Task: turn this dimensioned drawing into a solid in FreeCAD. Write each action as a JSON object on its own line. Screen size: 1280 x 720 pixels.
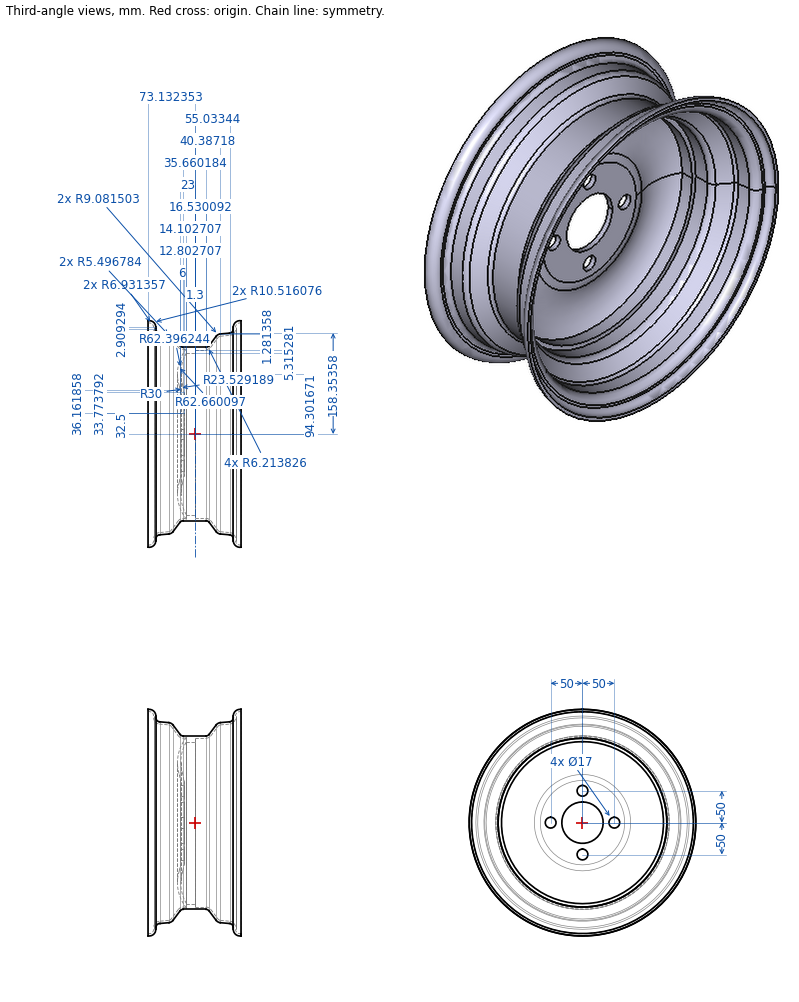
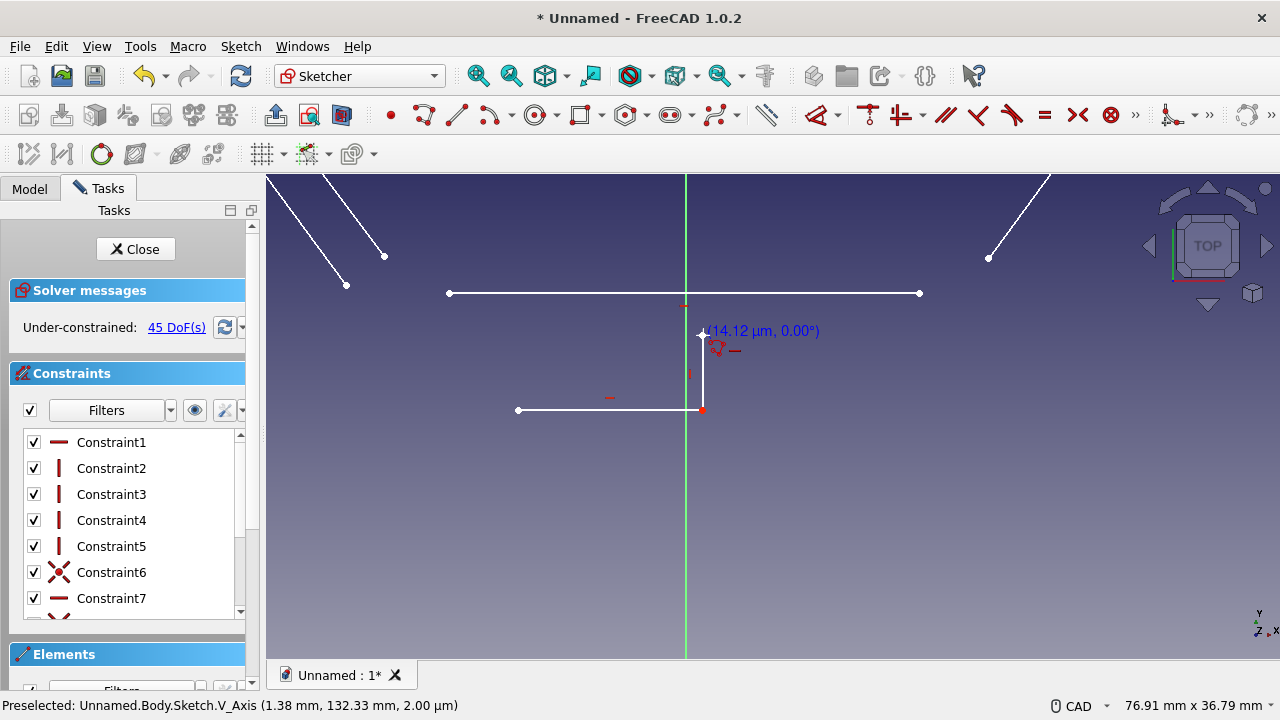
{"action": "scroll", "coordinate": [707, 339], "scroll_direction": "down", "scroll_amount": 10}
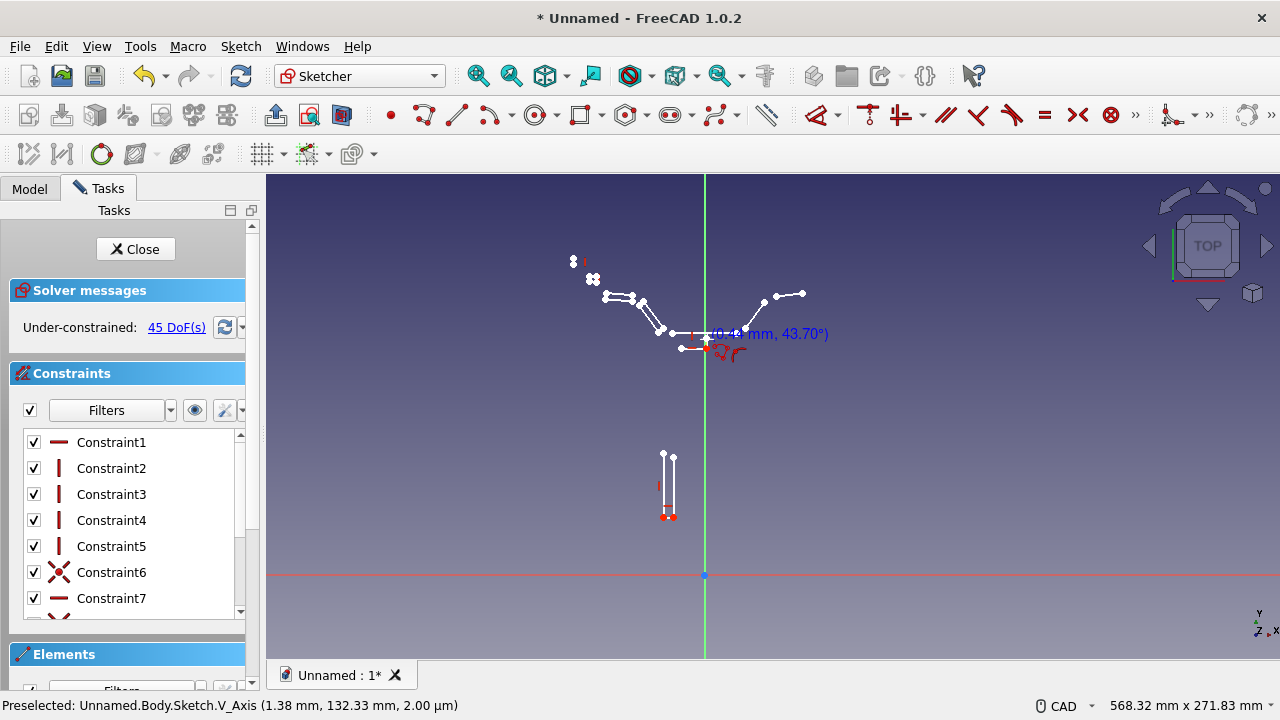
{"action": "scroll", "coordinate": [736, 339], "scroll_direction": "up", "scroll_amount": 5}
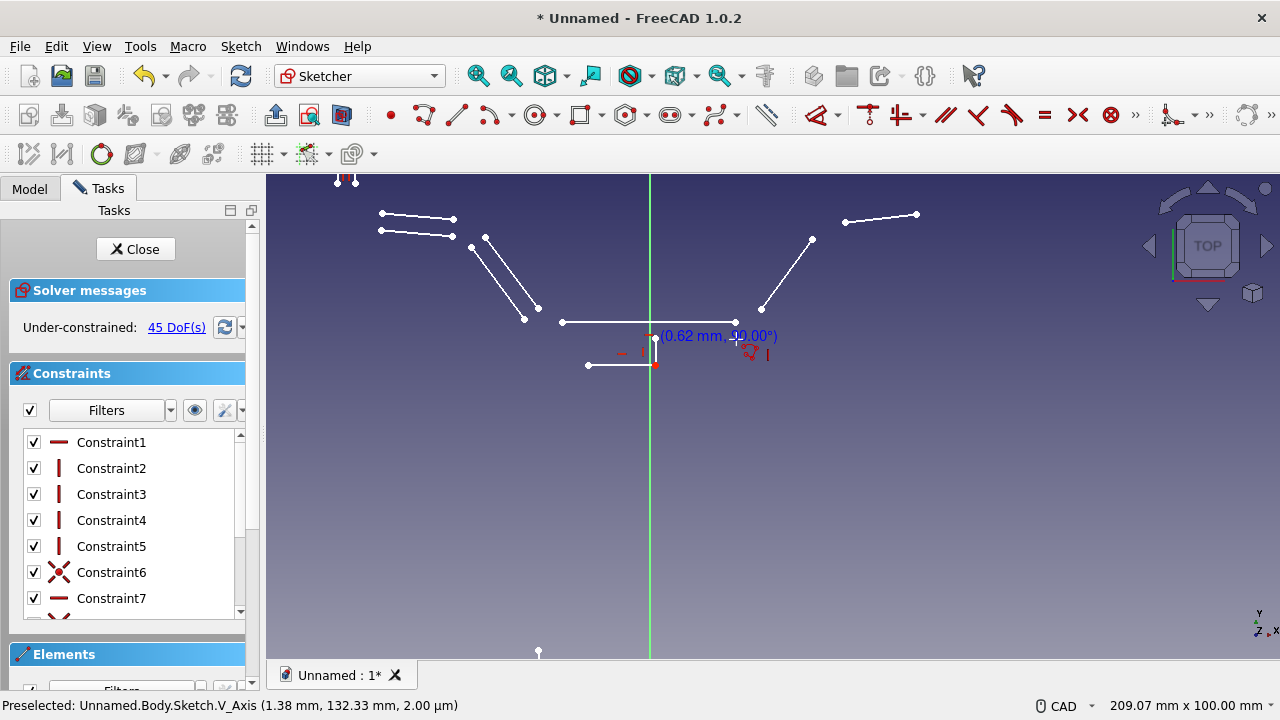
{"action": "left_click", "coordinate": [736, 338]}
{"action": "right_click", "coordinate": [736, 338]}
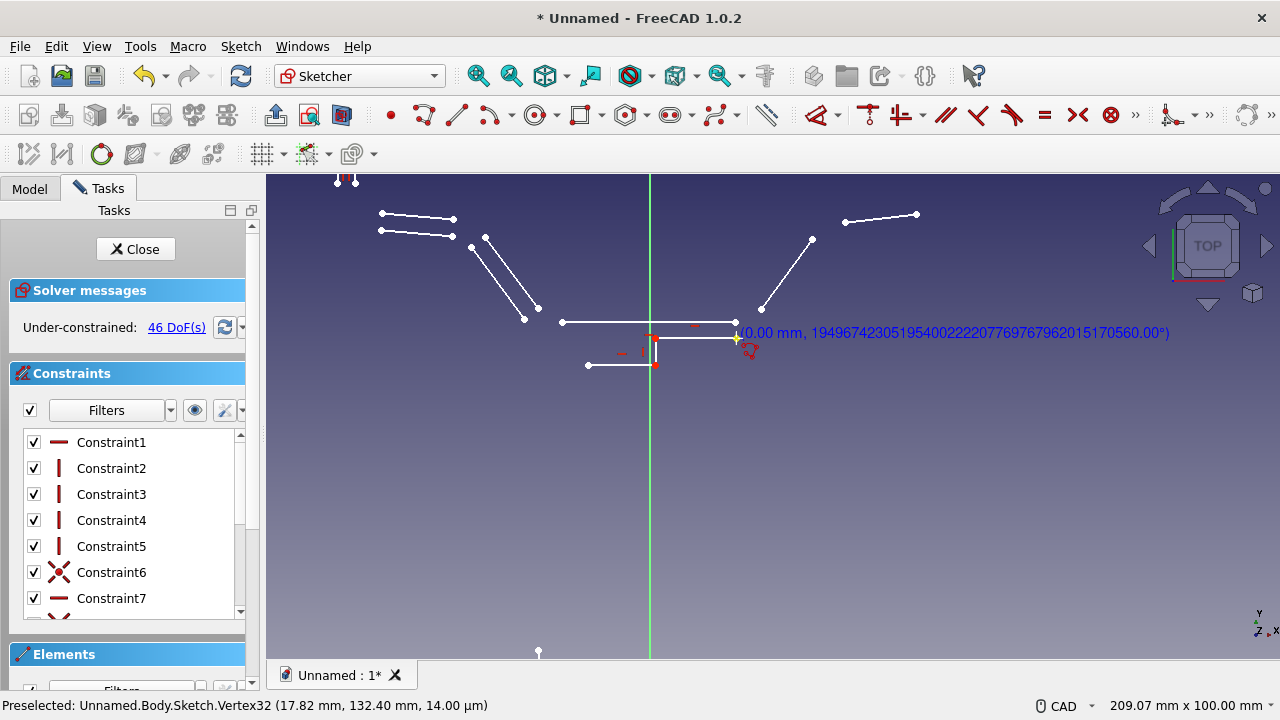
{"action": "left_click", "coordinate": [457, 116]}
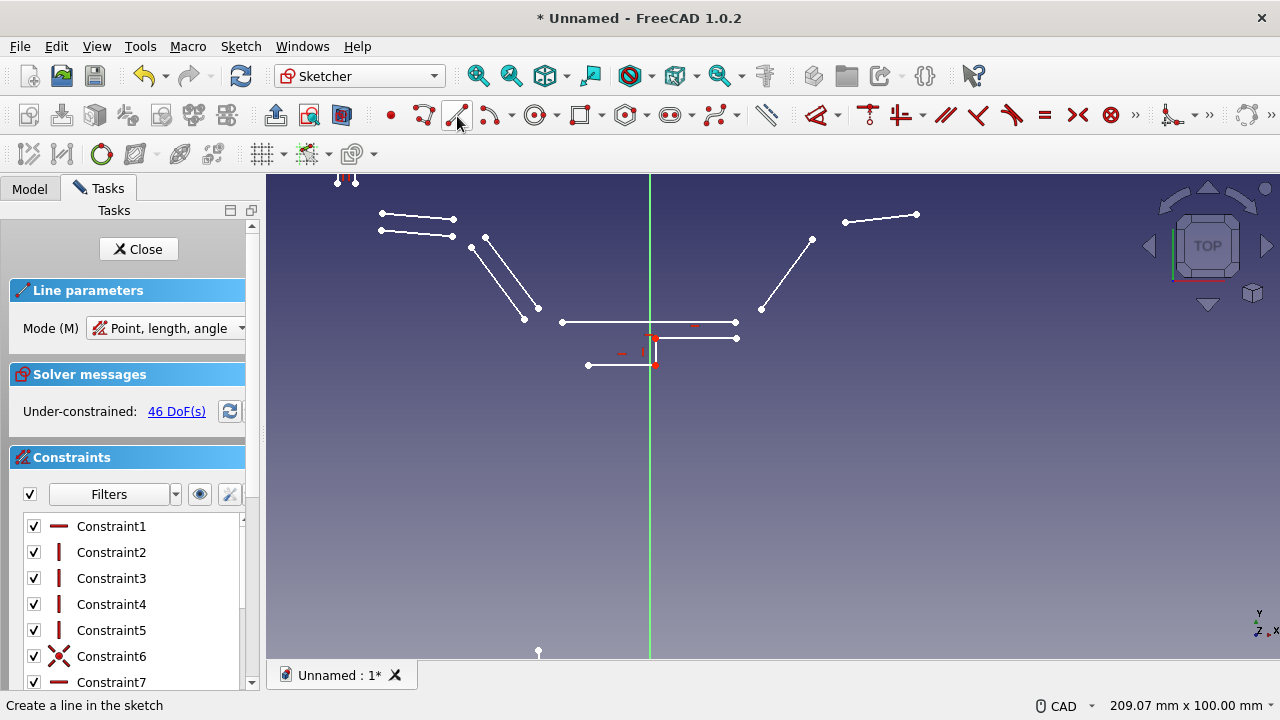
{"action": "left_click", "coordinate": [774, 318]}
{"action": "left_click", "coordinate": [828, 246]}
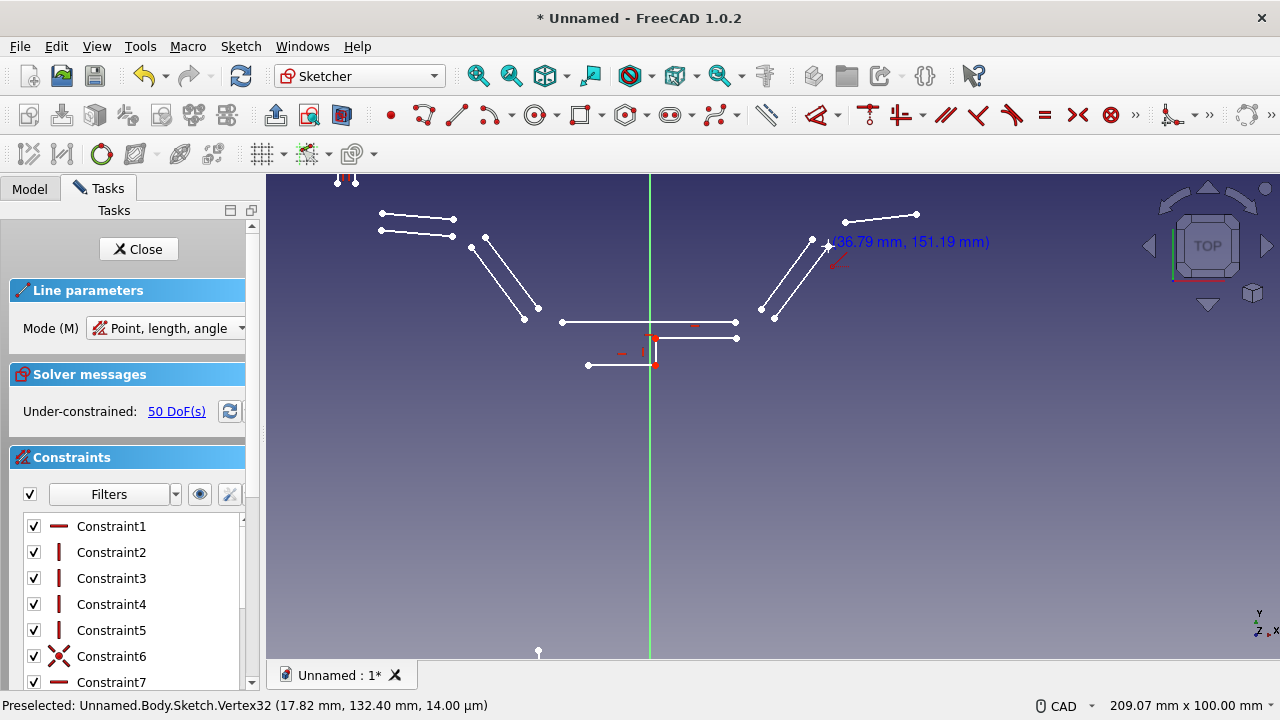
{"action": "left_click", "coordinate": [847, 236]}
{"action": "left_click", "coordinate": [918, 230]}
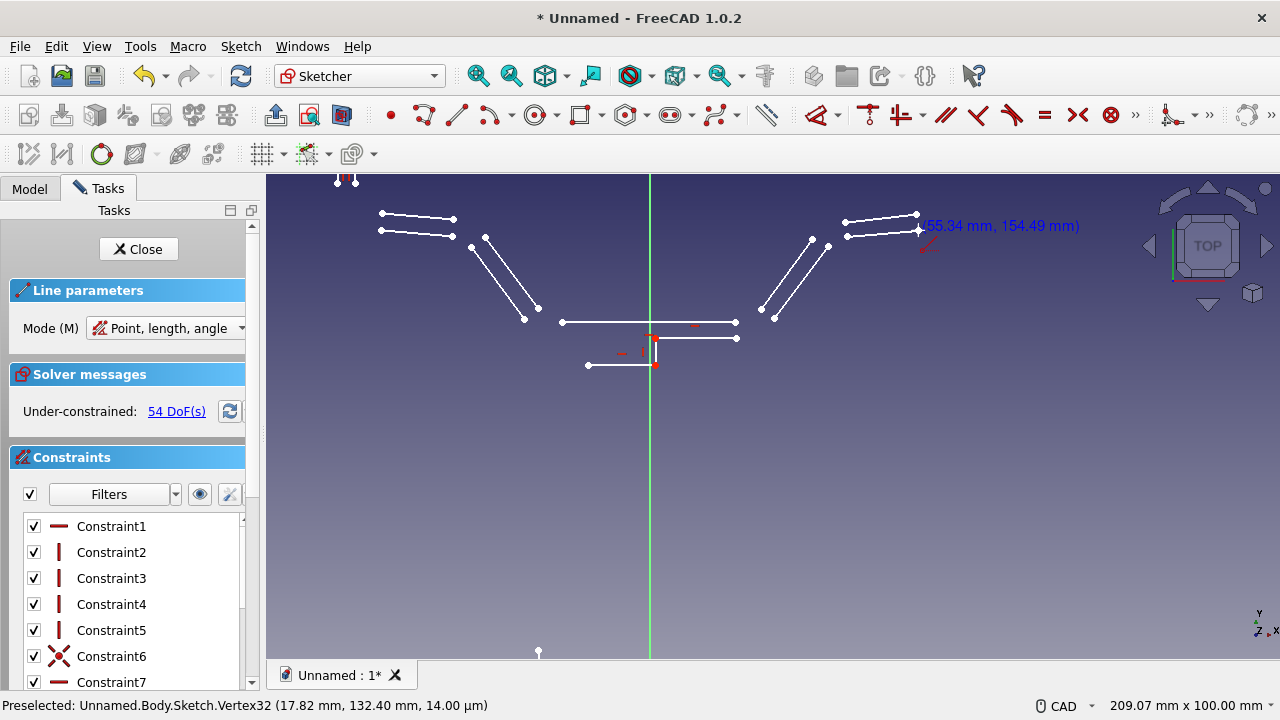
{"action": "scroll", "coordinate": [736, 339], "scroll_direction": "down", "scroll_amount": 5}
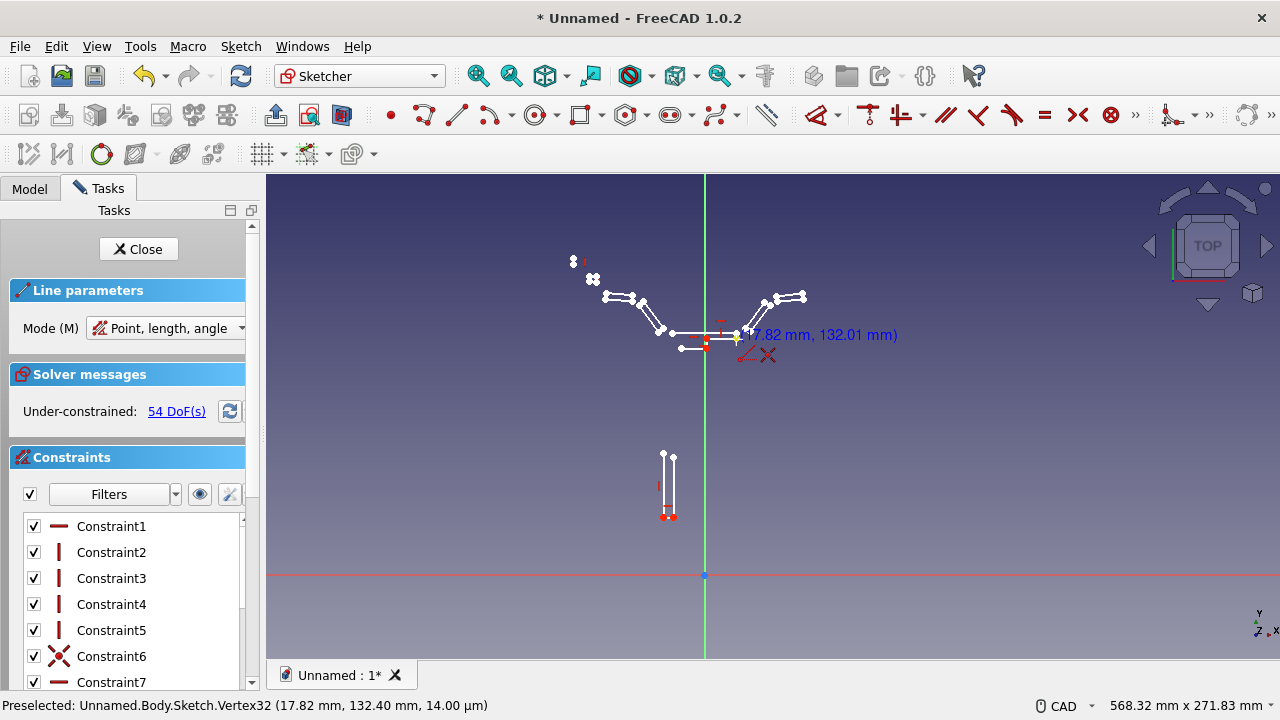
{"action": "left_click", "coordinate": [819, 282]}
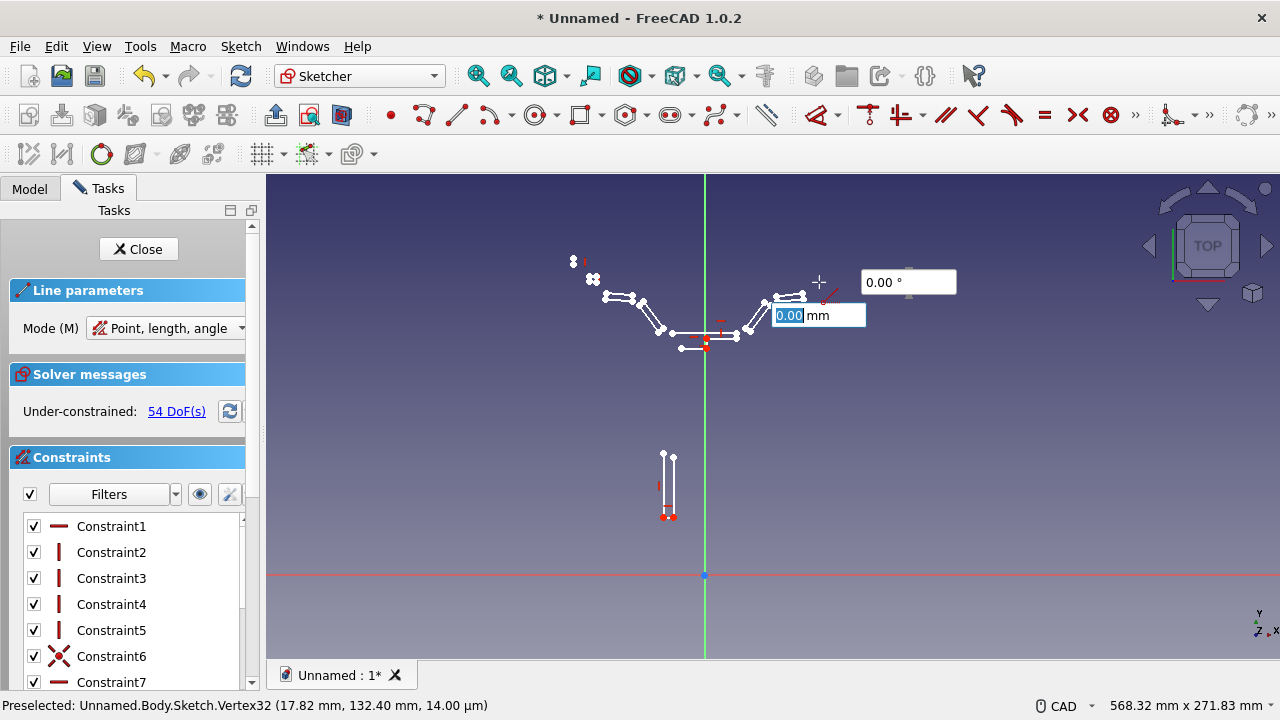
{"action": "scroll", "coordinate": [819, 276], "scroll_direction": "up", "scroll_amount": 6}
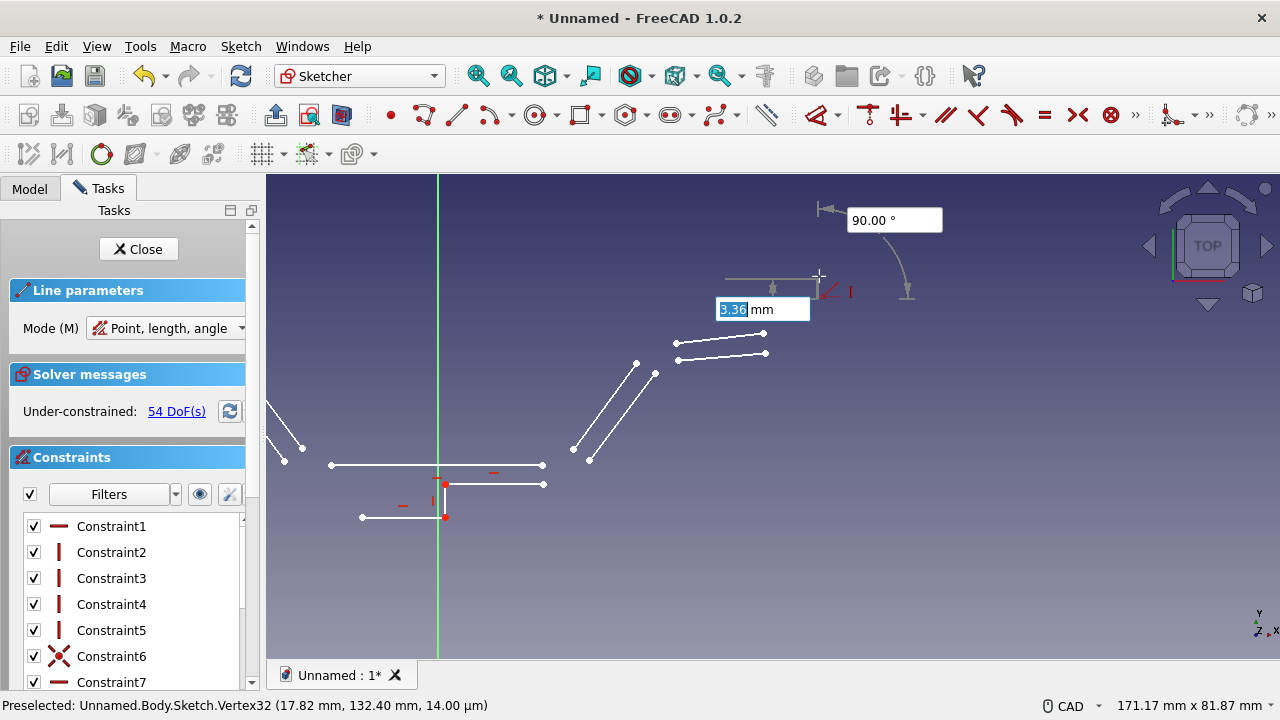
{"action": "left_click", "coordinate": [818, 277]}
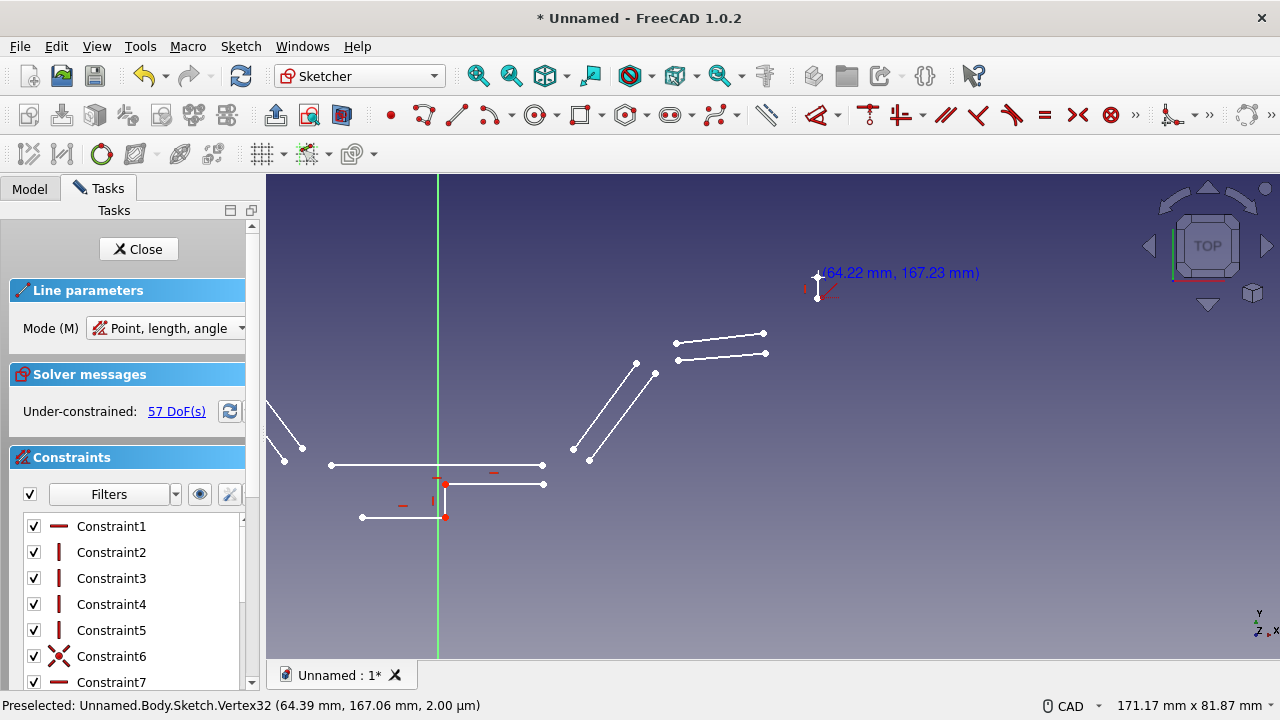
{"action": "left_click", "coordinate": [871, 237]}
{"action": "left_click", "coordinate": [871, 215]}